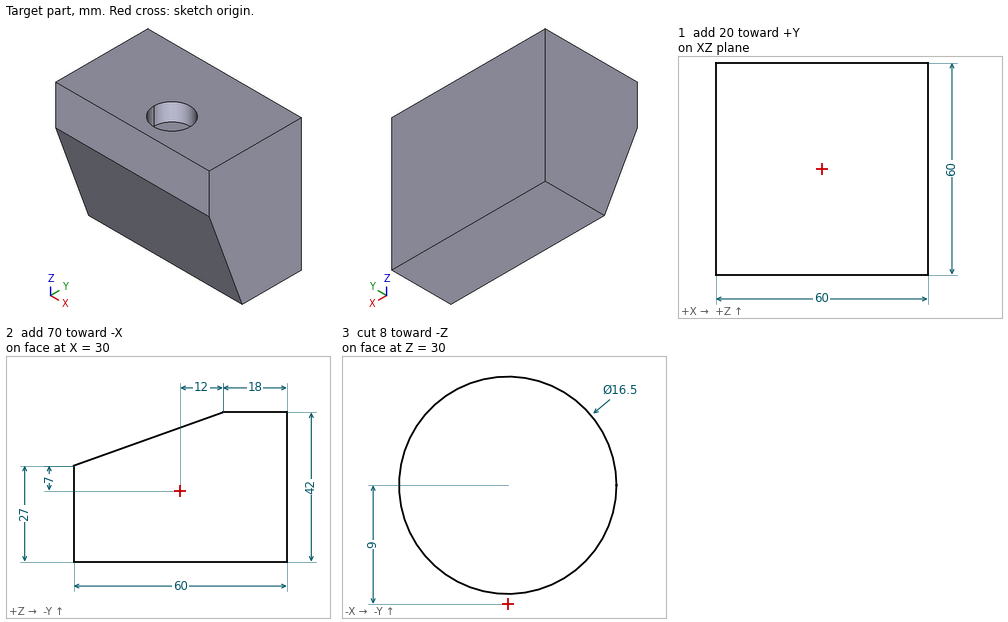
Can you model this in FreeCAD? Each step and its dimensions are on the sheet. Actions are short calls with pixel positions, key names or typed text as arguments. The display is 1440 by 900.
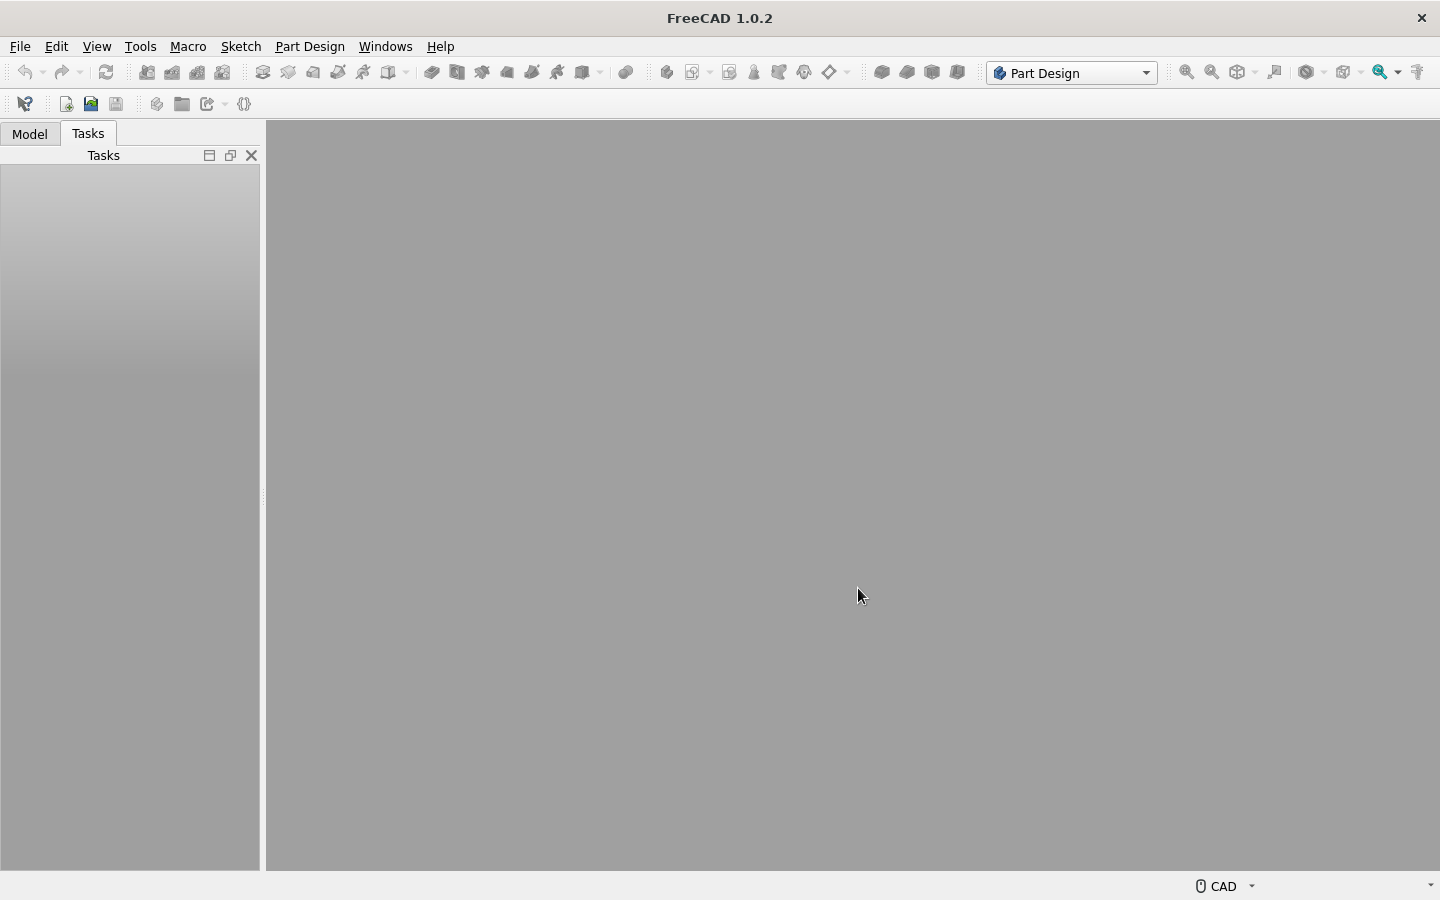
click(66, 104)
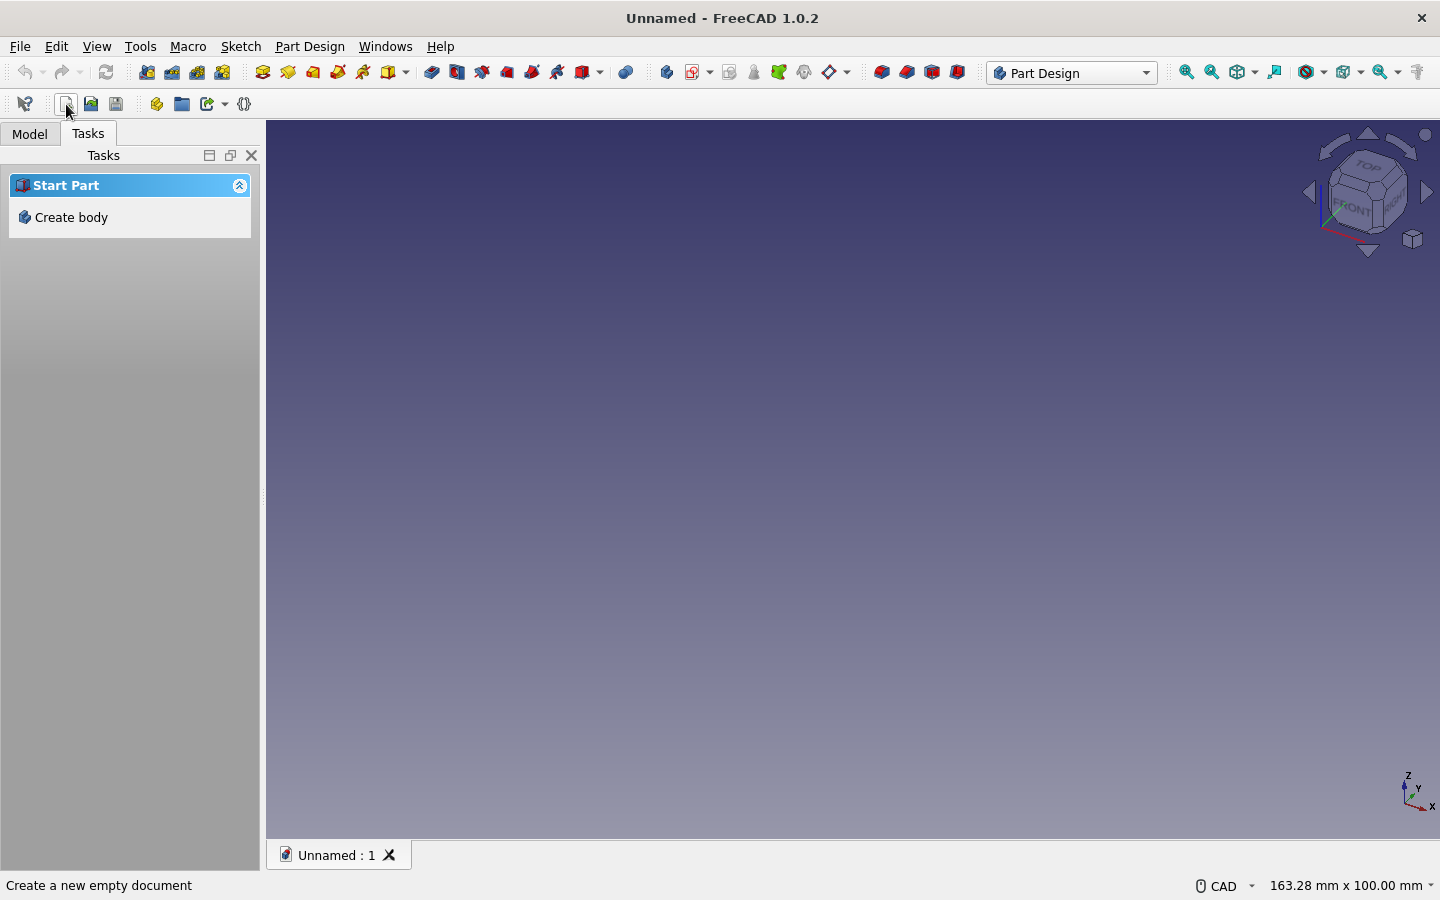
click(692, 72)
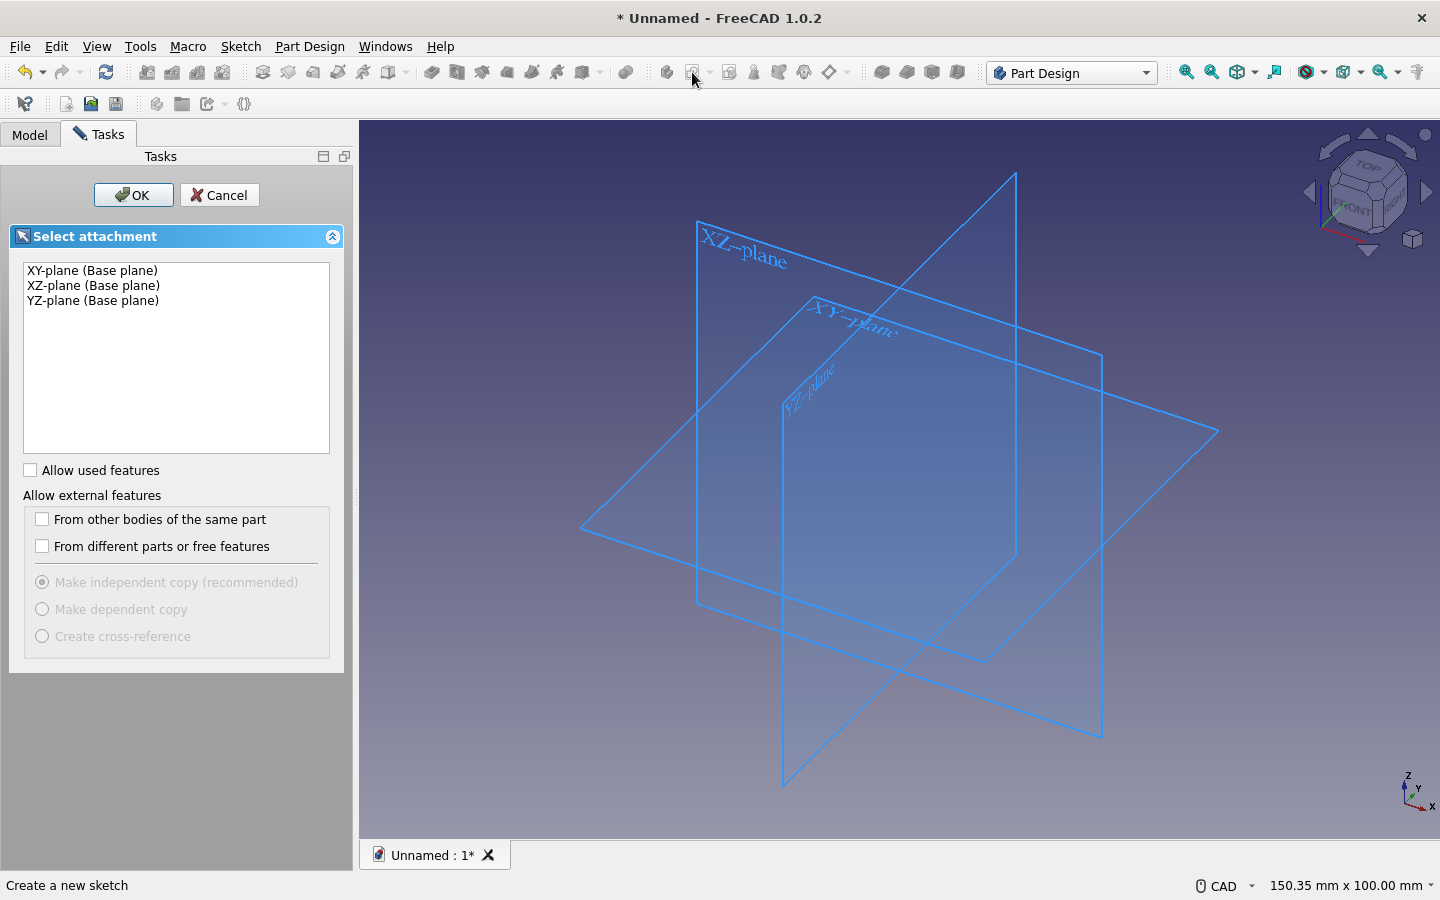
click(84, 286)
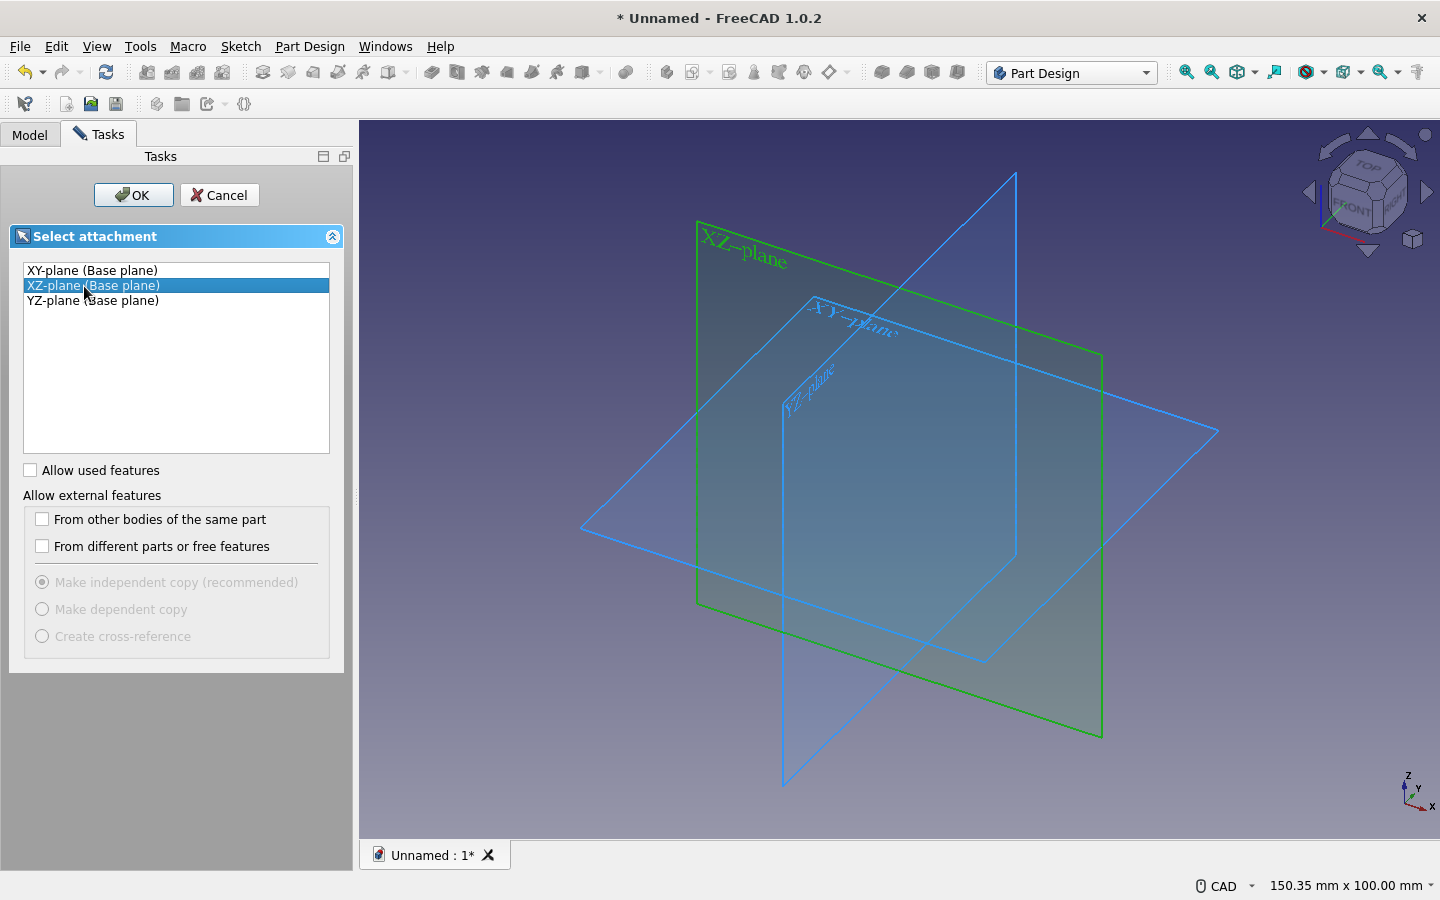
click(134, 195)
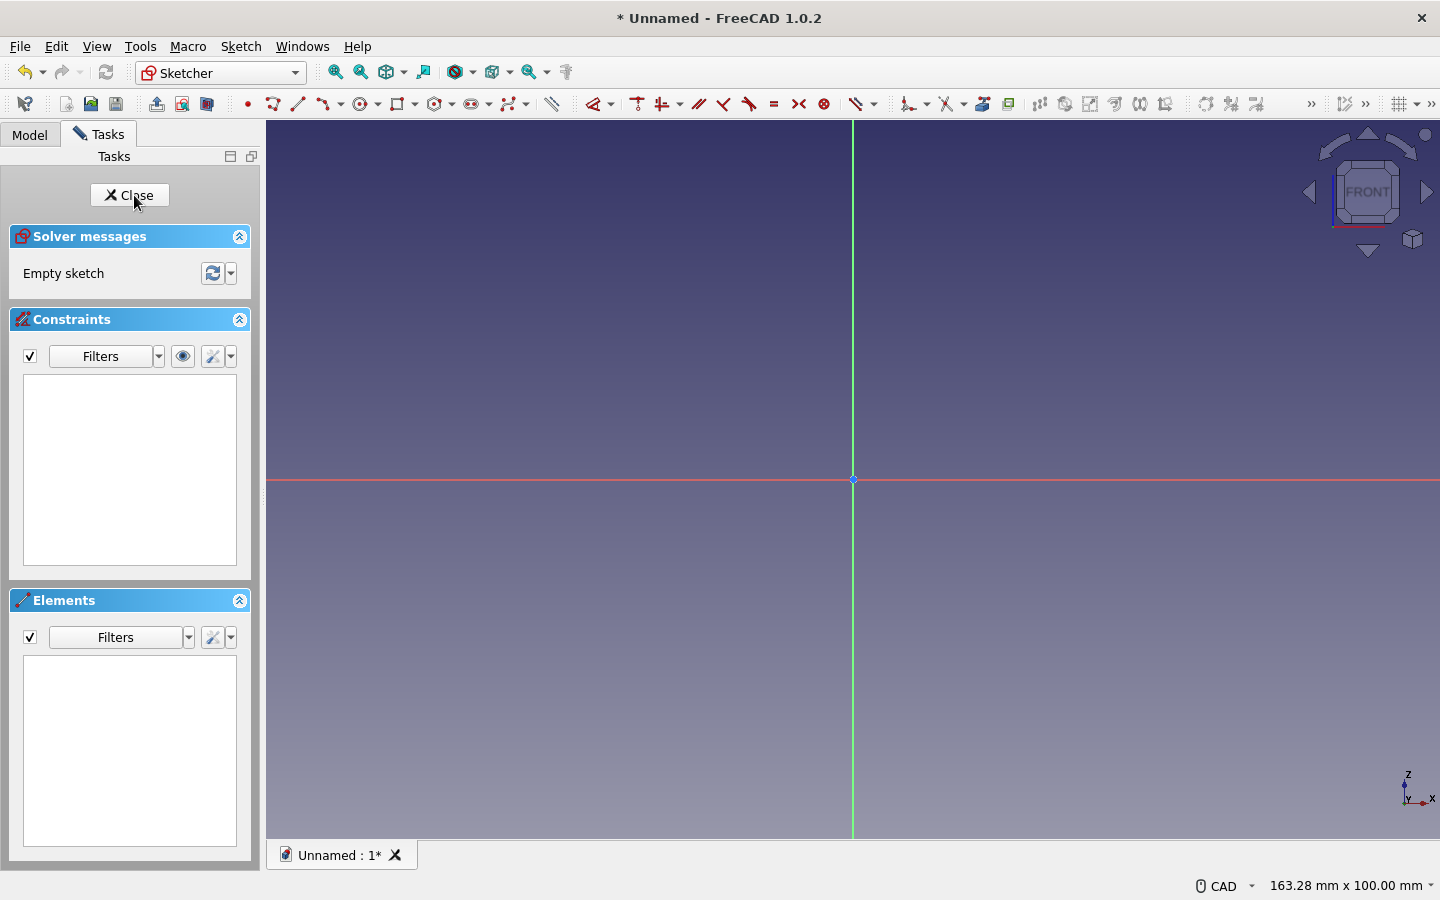
click(414, 104)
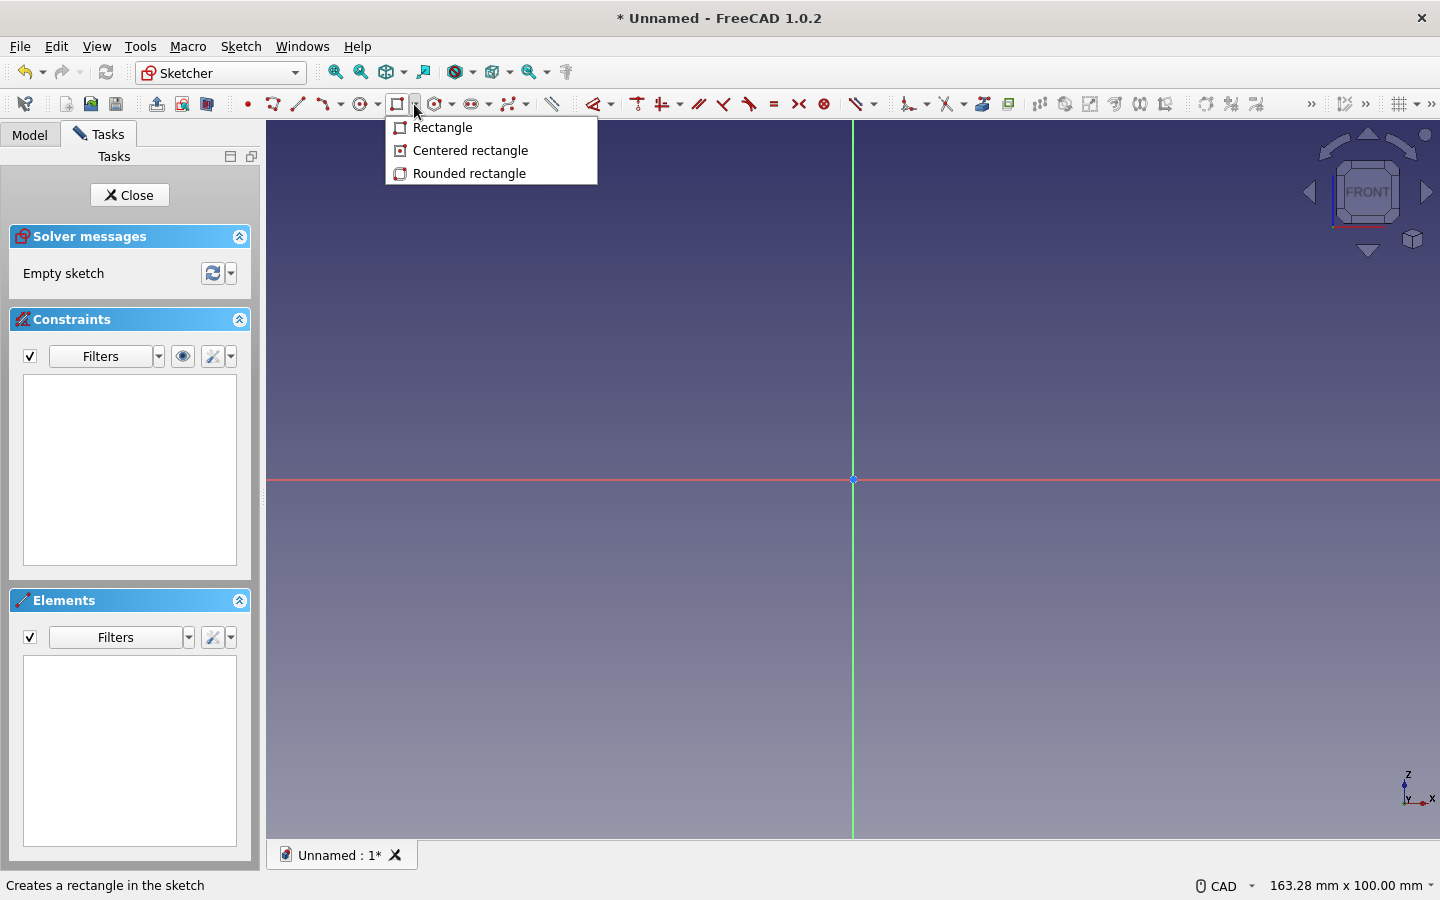
click(492, 150)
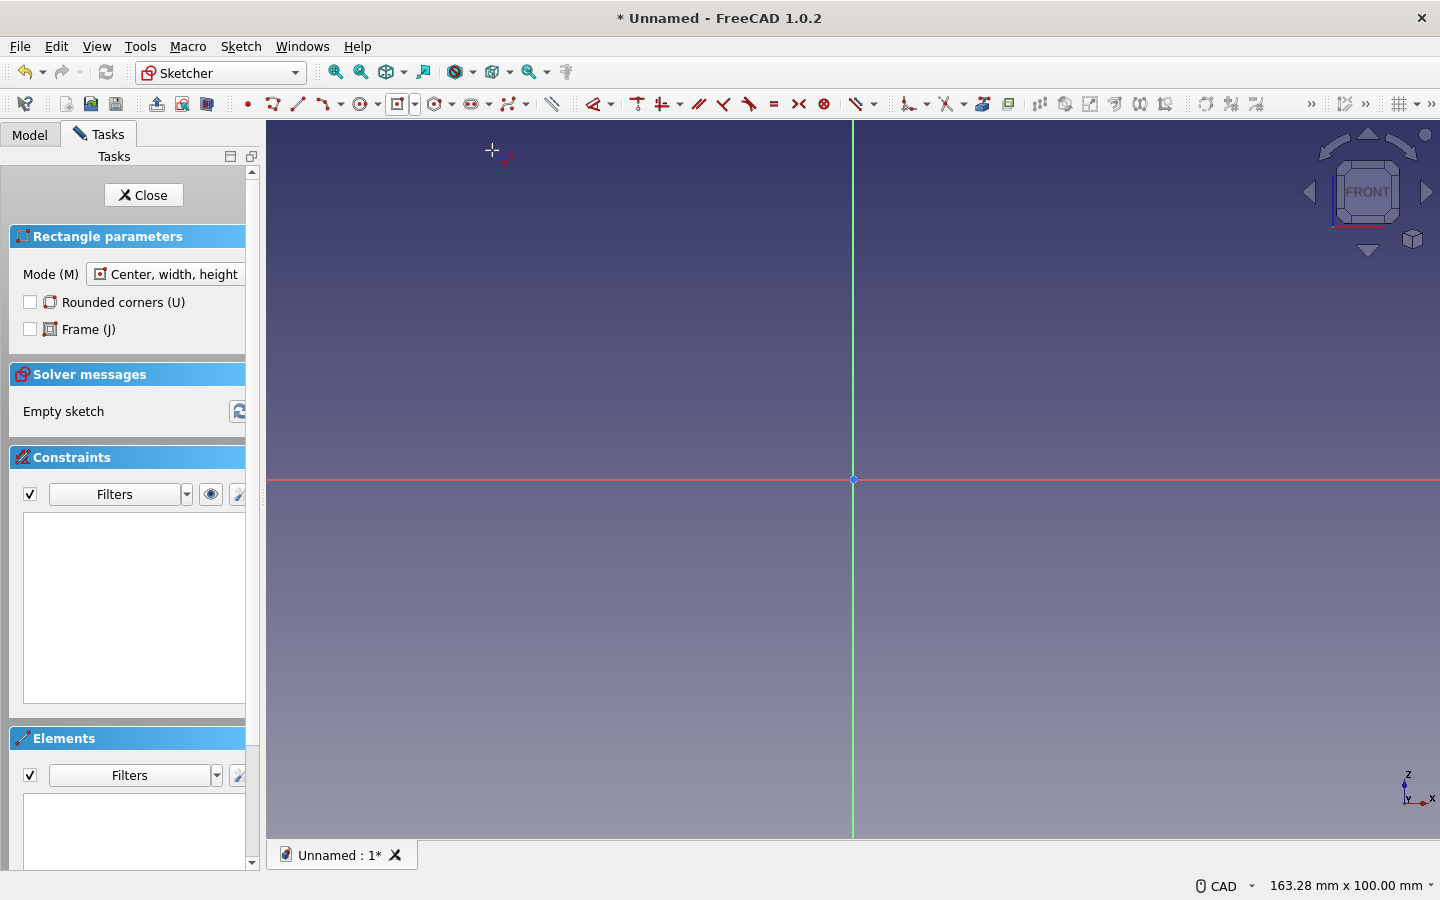
click(853, 480)
click(1069, 264)
key(Escape)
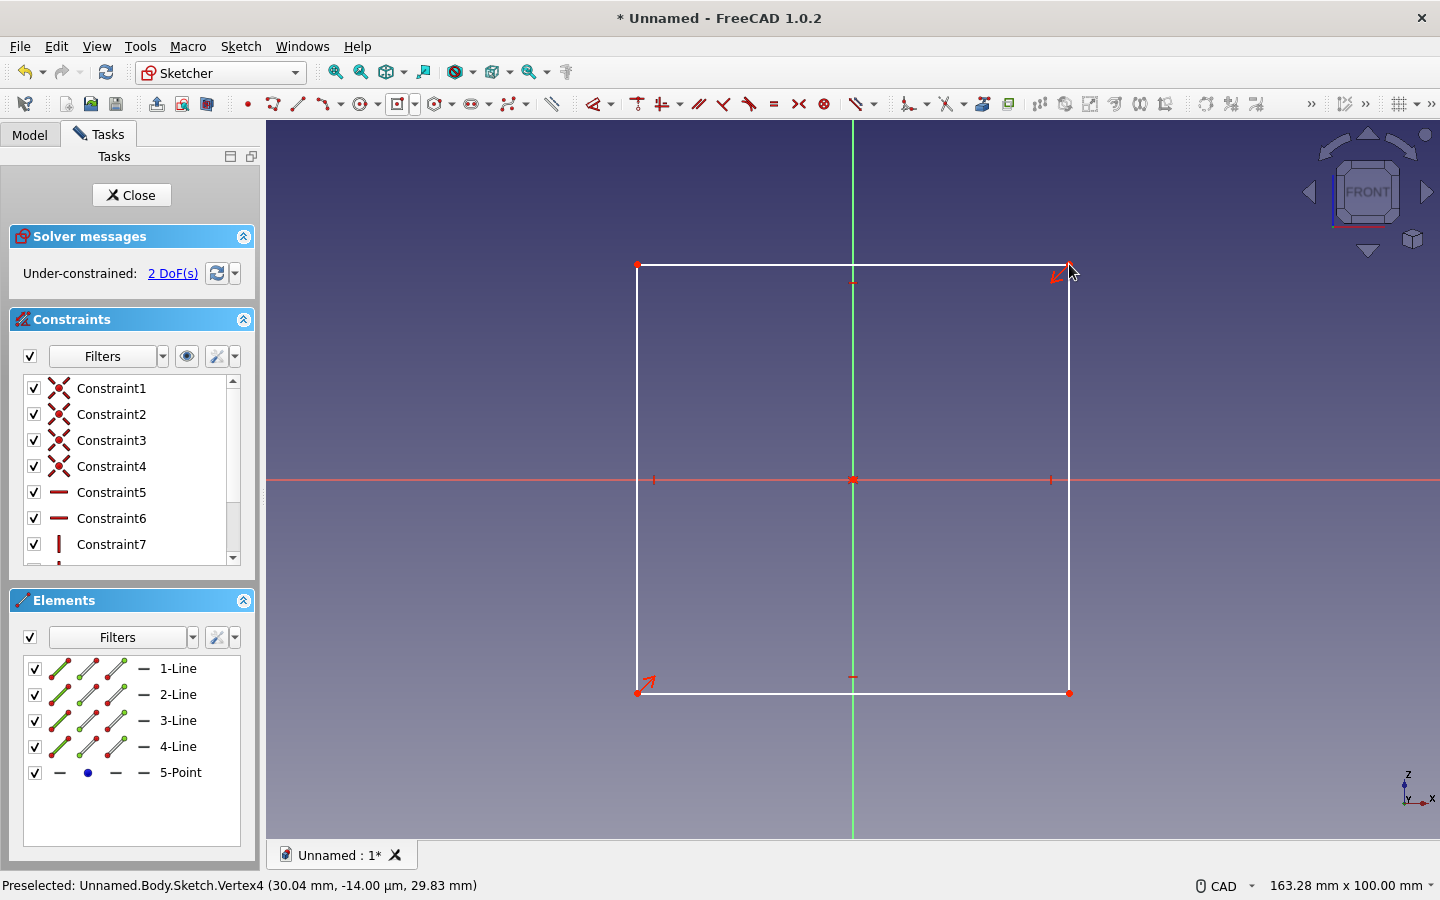
click(592, 104)